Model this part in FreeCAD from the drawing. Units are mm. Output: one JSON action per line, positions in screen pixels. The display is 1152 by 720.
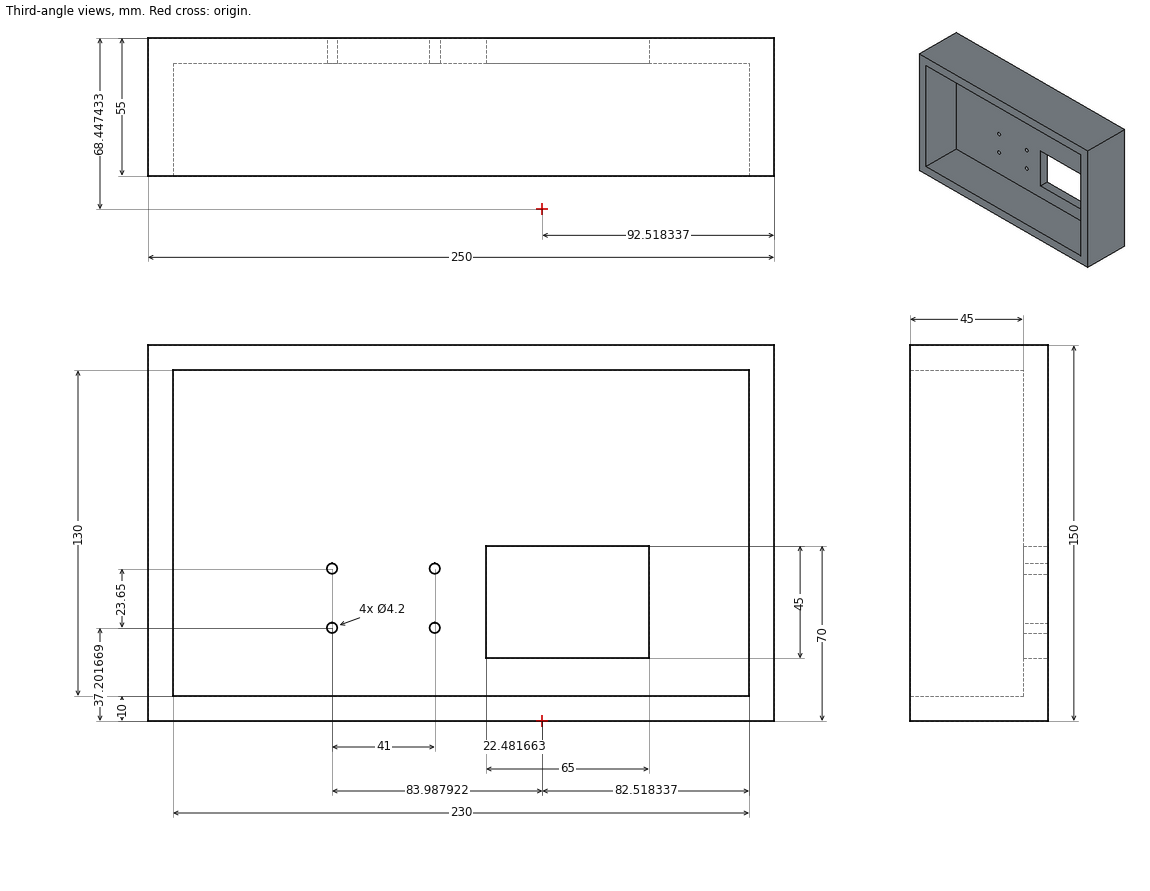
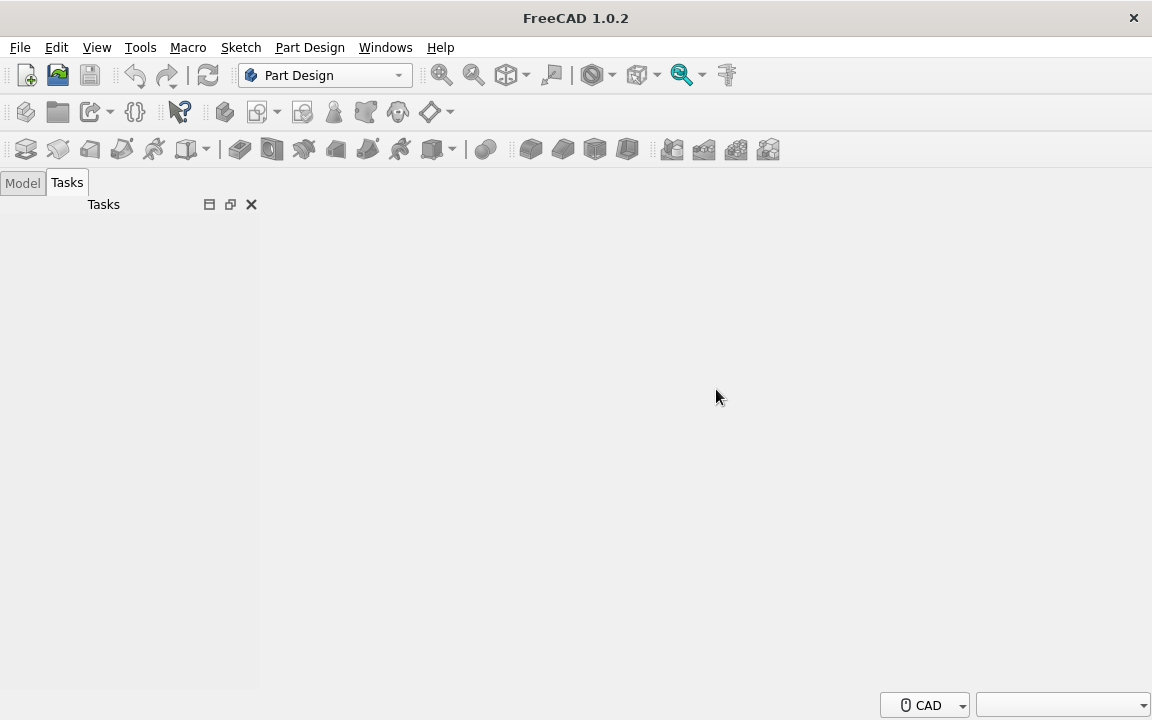
{"action": "left_click", "coordinate": [26, 76]}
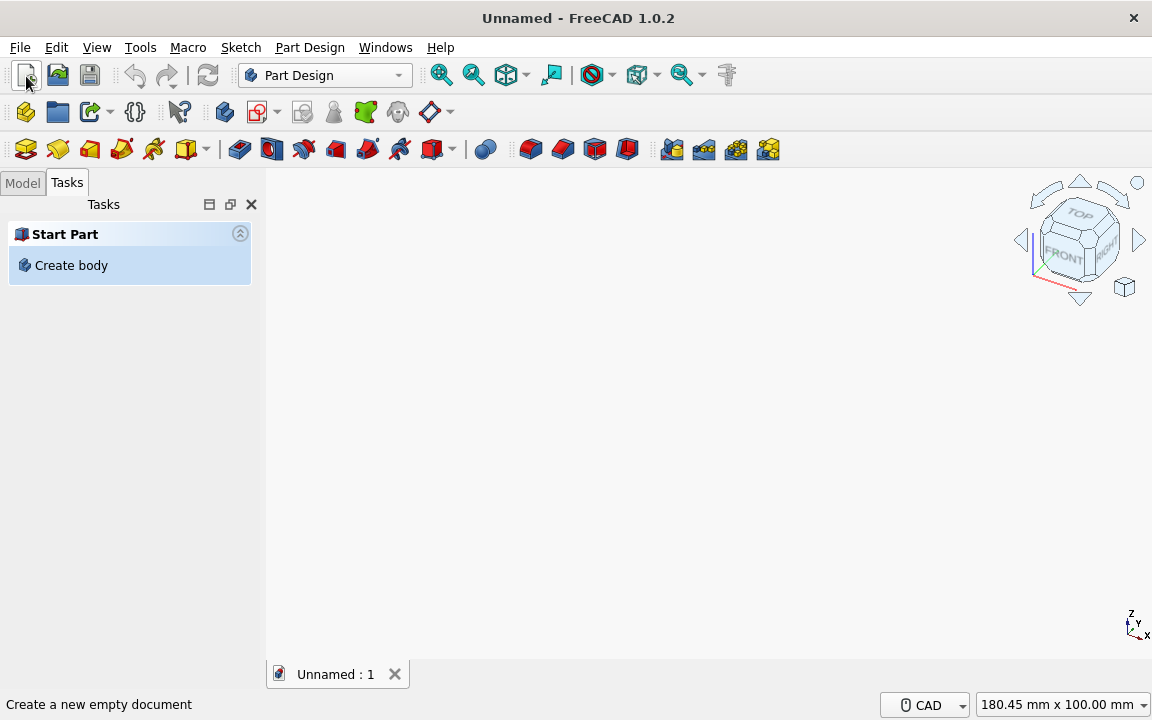
{"action": "left_click", "coordinate": [258, 112]}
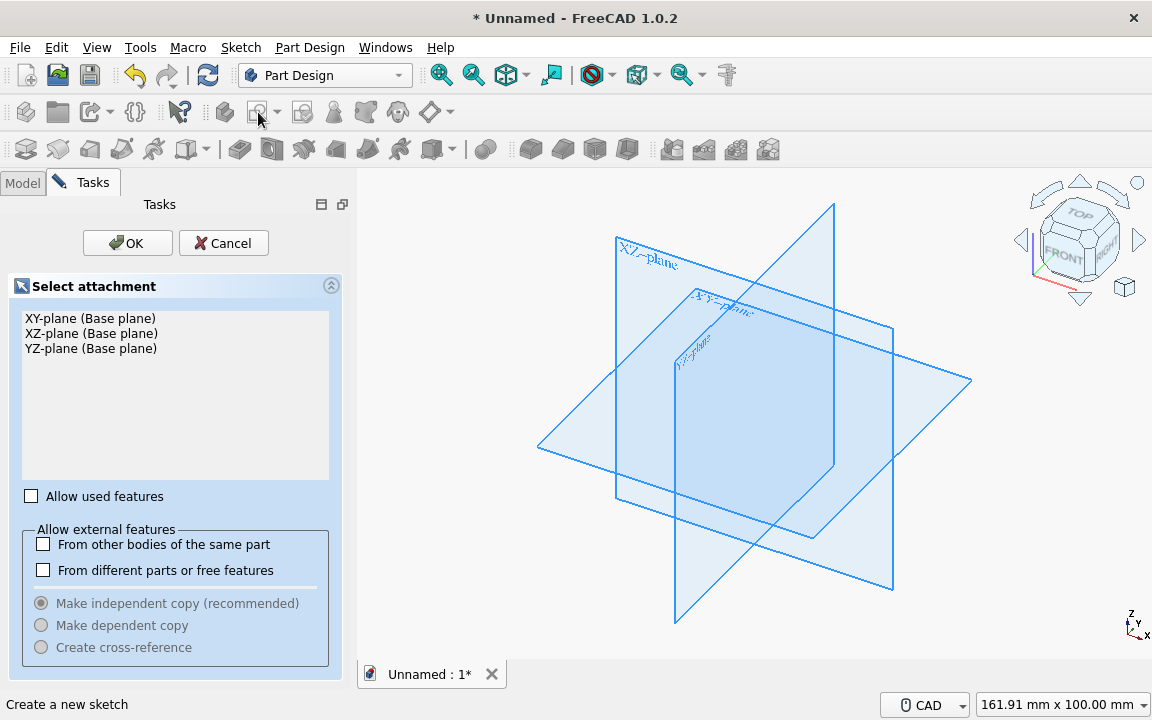
{"action": "left_click", "coordinate": [82, 318]}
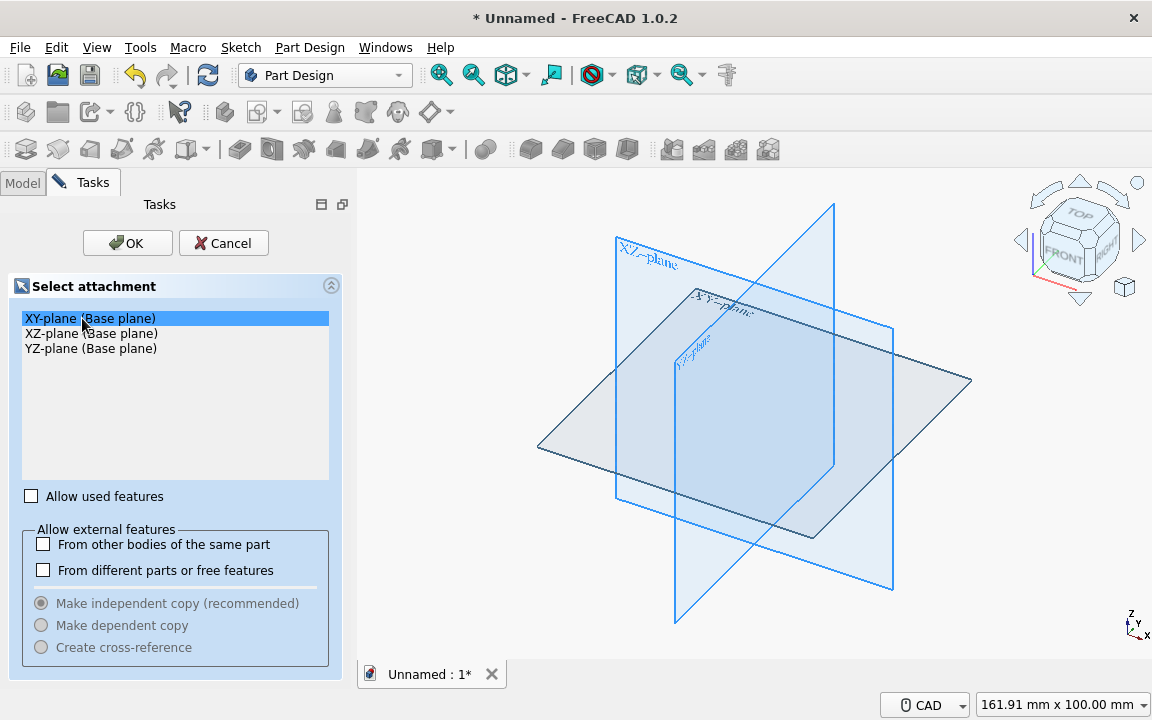
{"action": "left_click", "coordinate": [128, 243]}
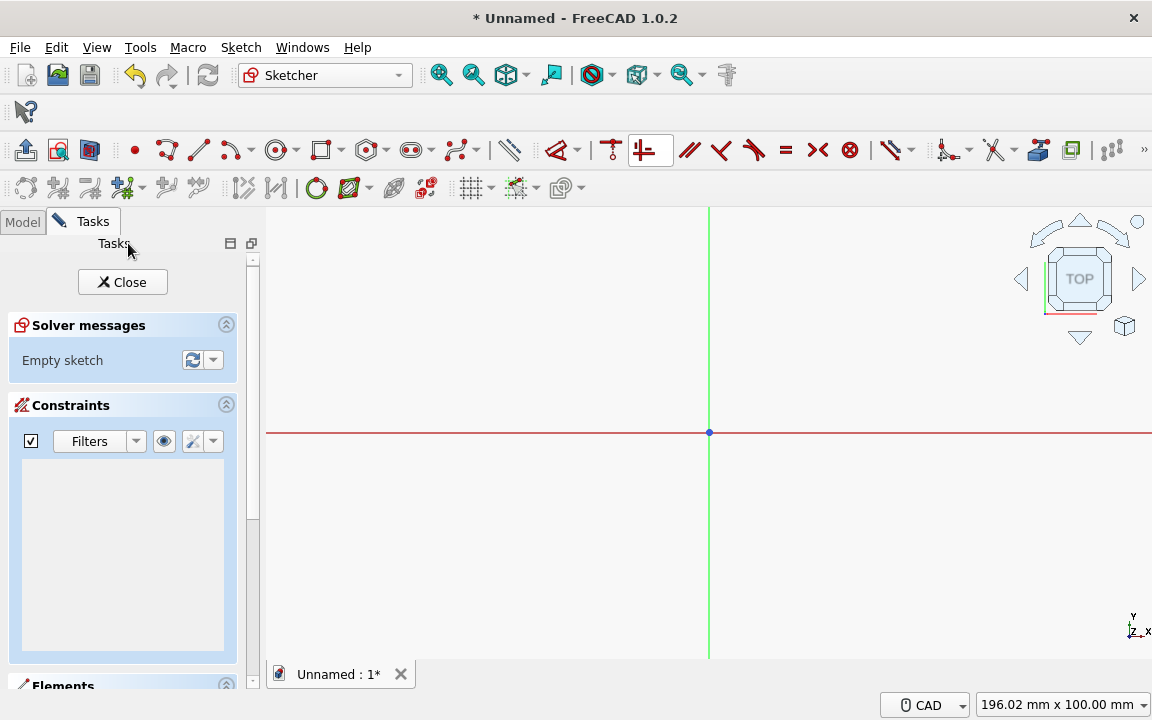
{"action": "scroll", "coordinate": [704, 559], "scroll_direction": "down", "scroll_amount": 4}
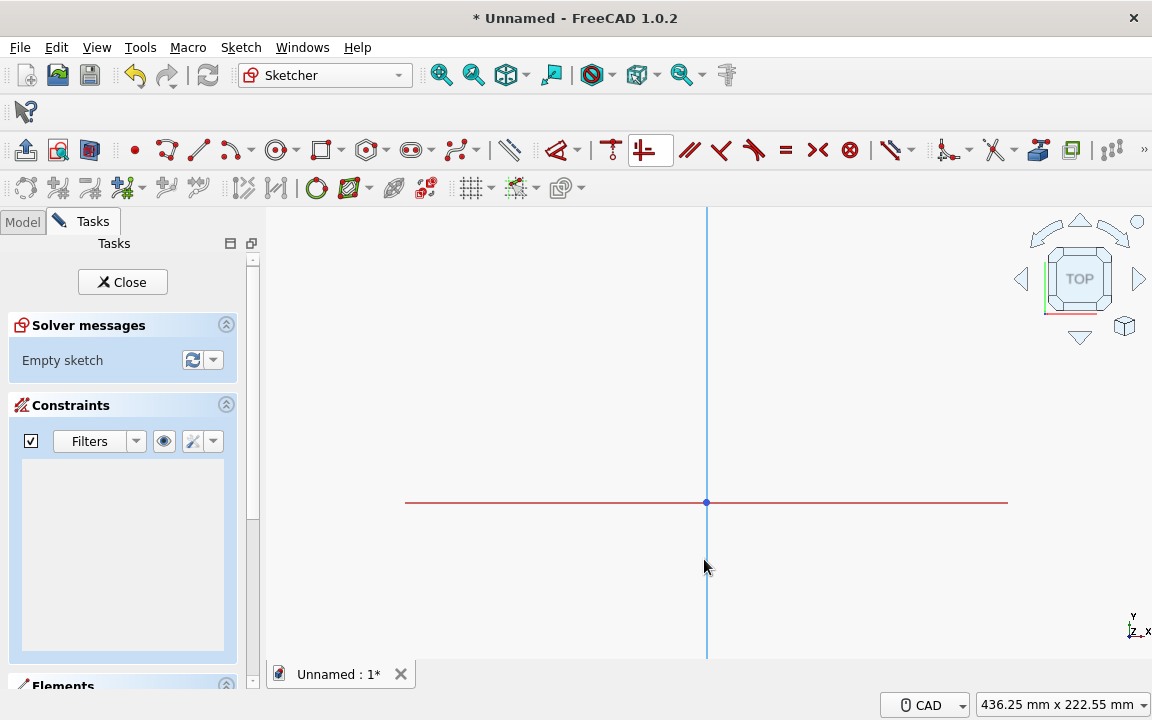
{"action": "left_click", "coordinate": [322, 150]}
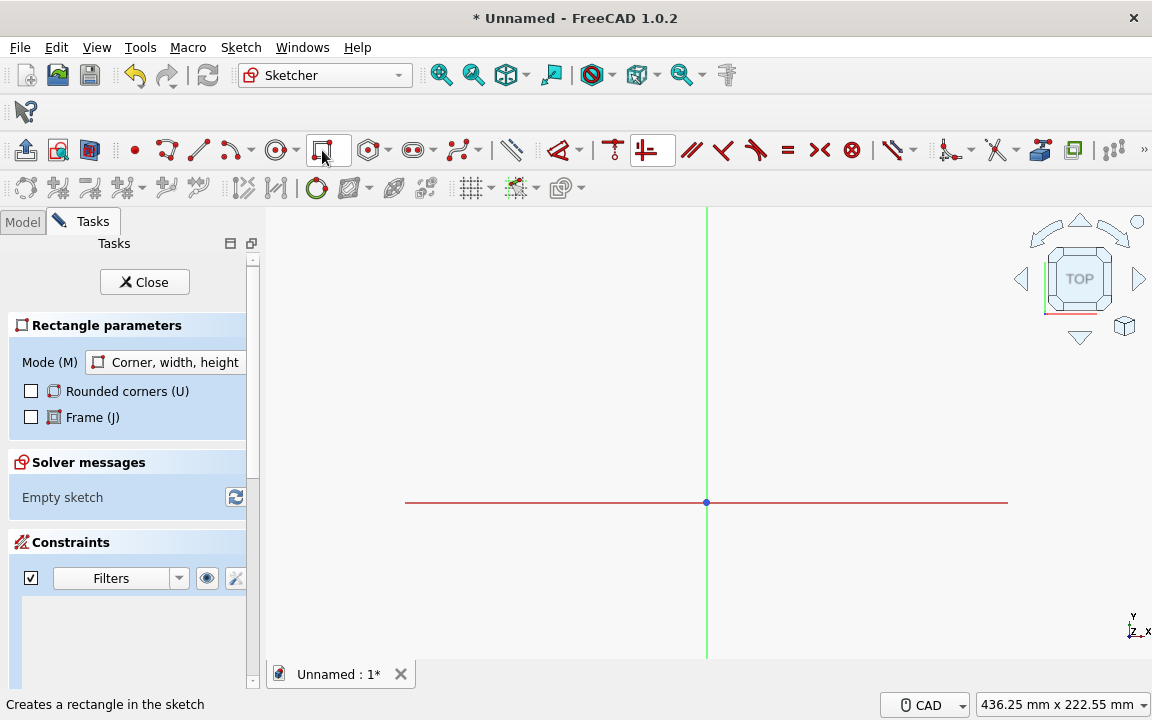
{"action": "left_click", "coordinate": [387, 364]}
{"action": "left_click", "coordinate": [894, 476]}
{"action": "key", "text": "Escape"}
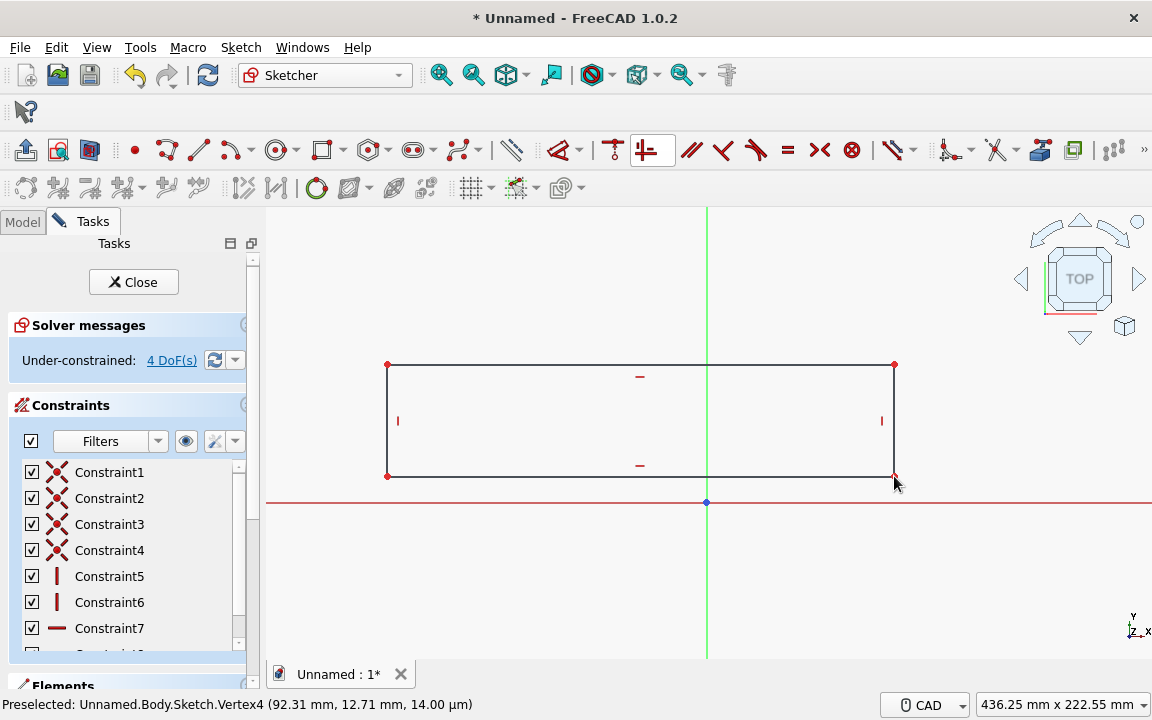
{"action": "left_click", "coordinate": [558, 150]}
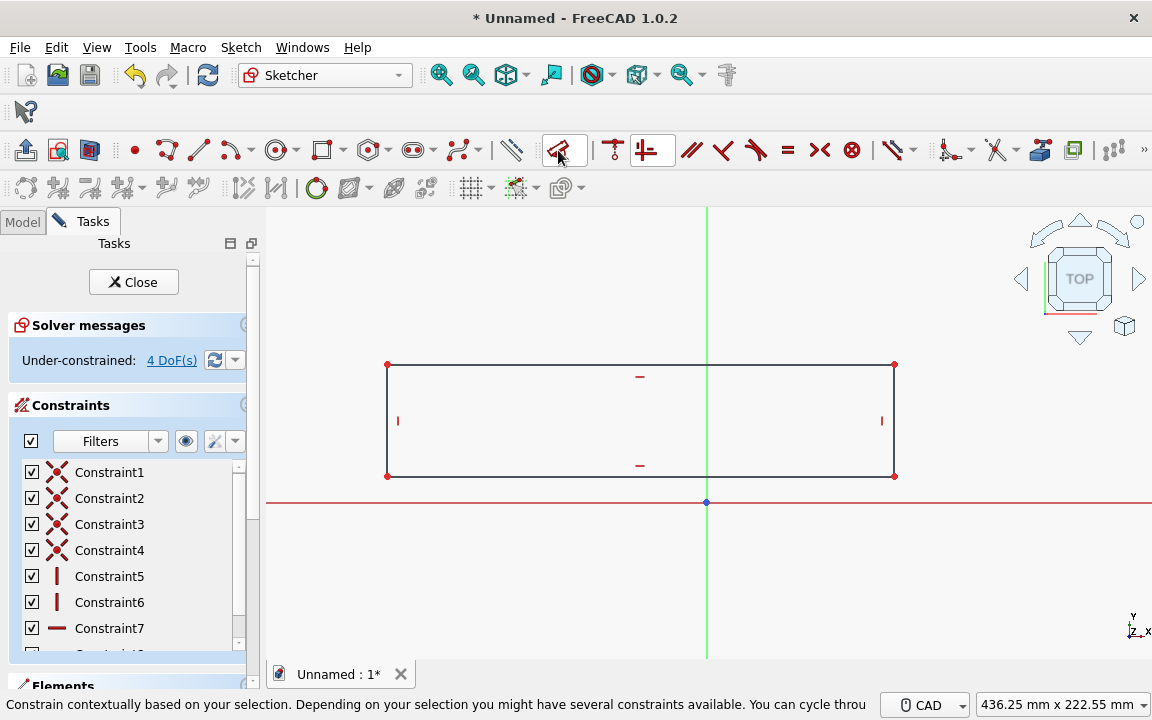
{"action": "left_click", "coordinate": [387, 399]}
{"action": "left_click", "coordinate": [353, 421]}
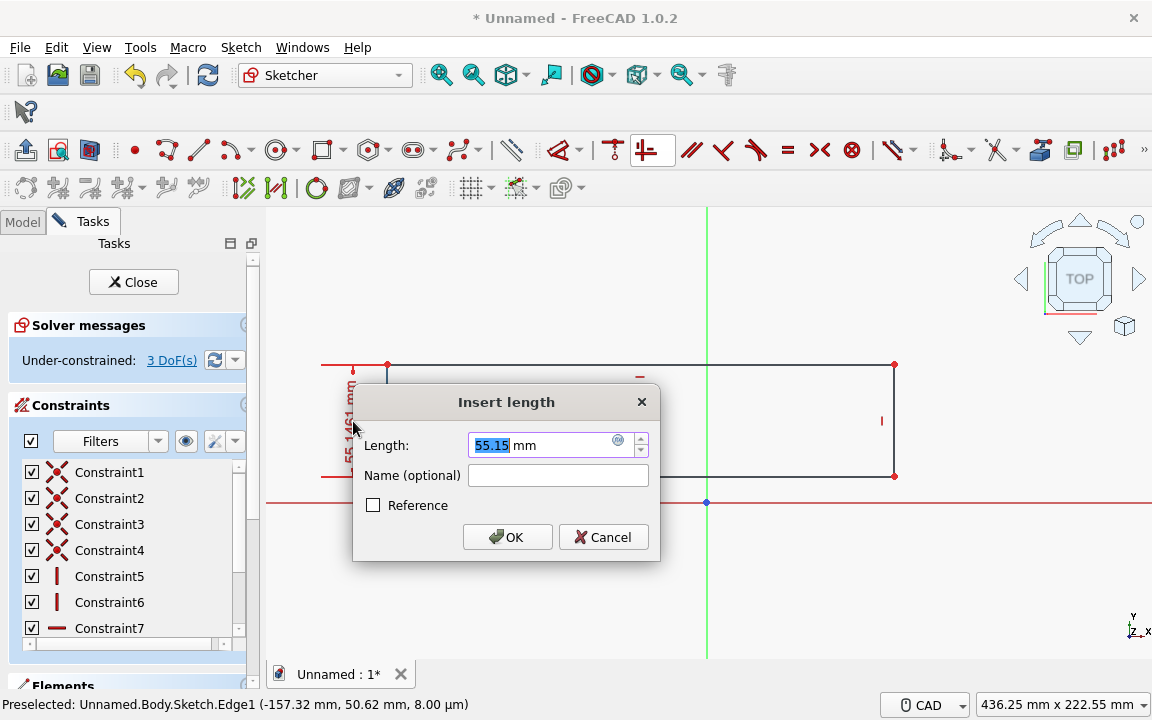
{"action": "type", "text": "55"}
{"action": "key", "text": "Return"}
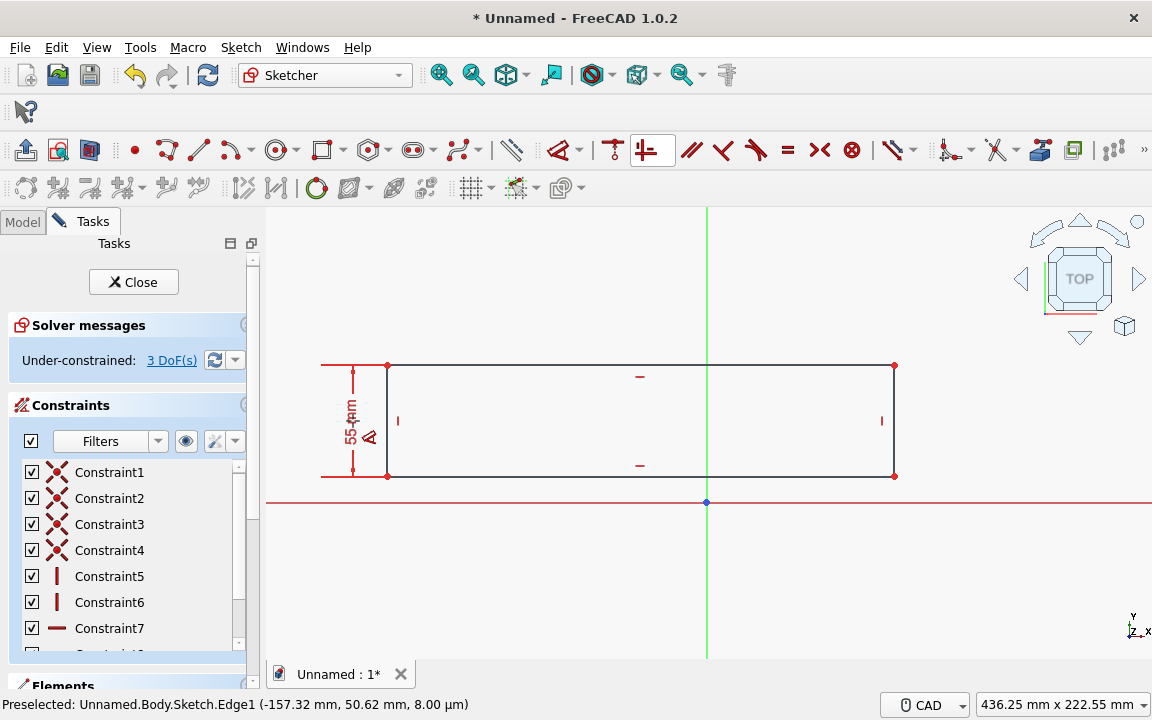
{"action": "left_click", "coordinate": [539, 477]}
{"action": "left_click", "coordinate": [640, 443]}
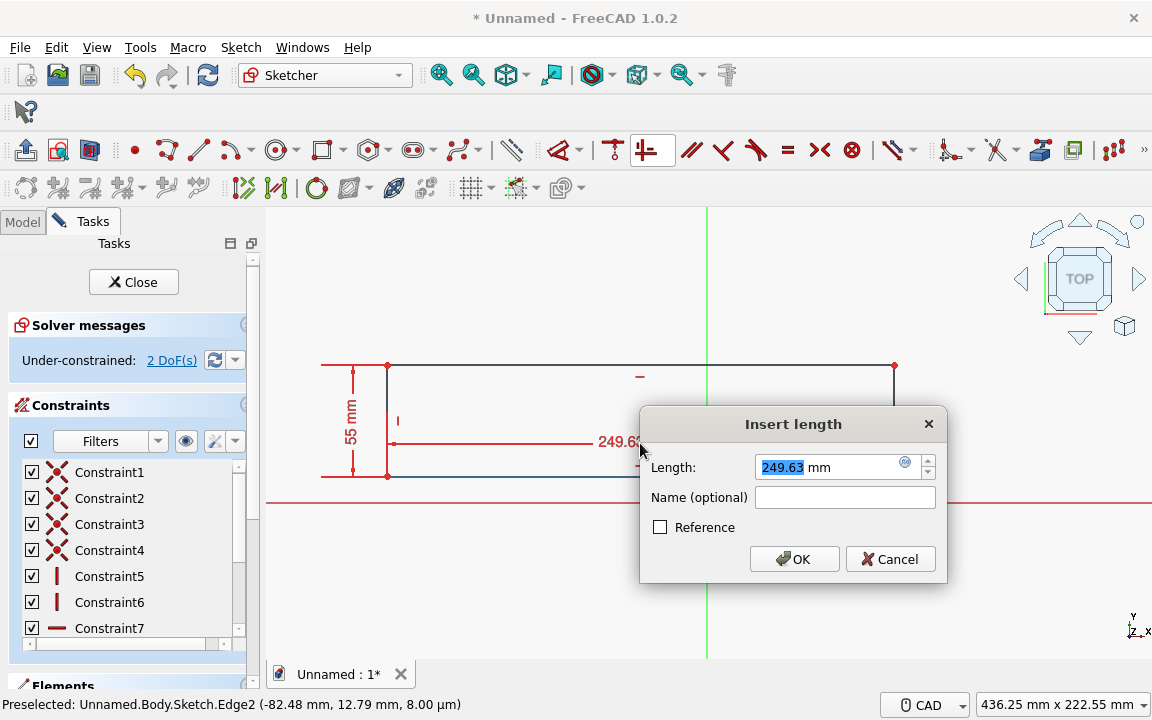
{"action": "type", "text": "250"}
{"action": "key", "text": "Return"}